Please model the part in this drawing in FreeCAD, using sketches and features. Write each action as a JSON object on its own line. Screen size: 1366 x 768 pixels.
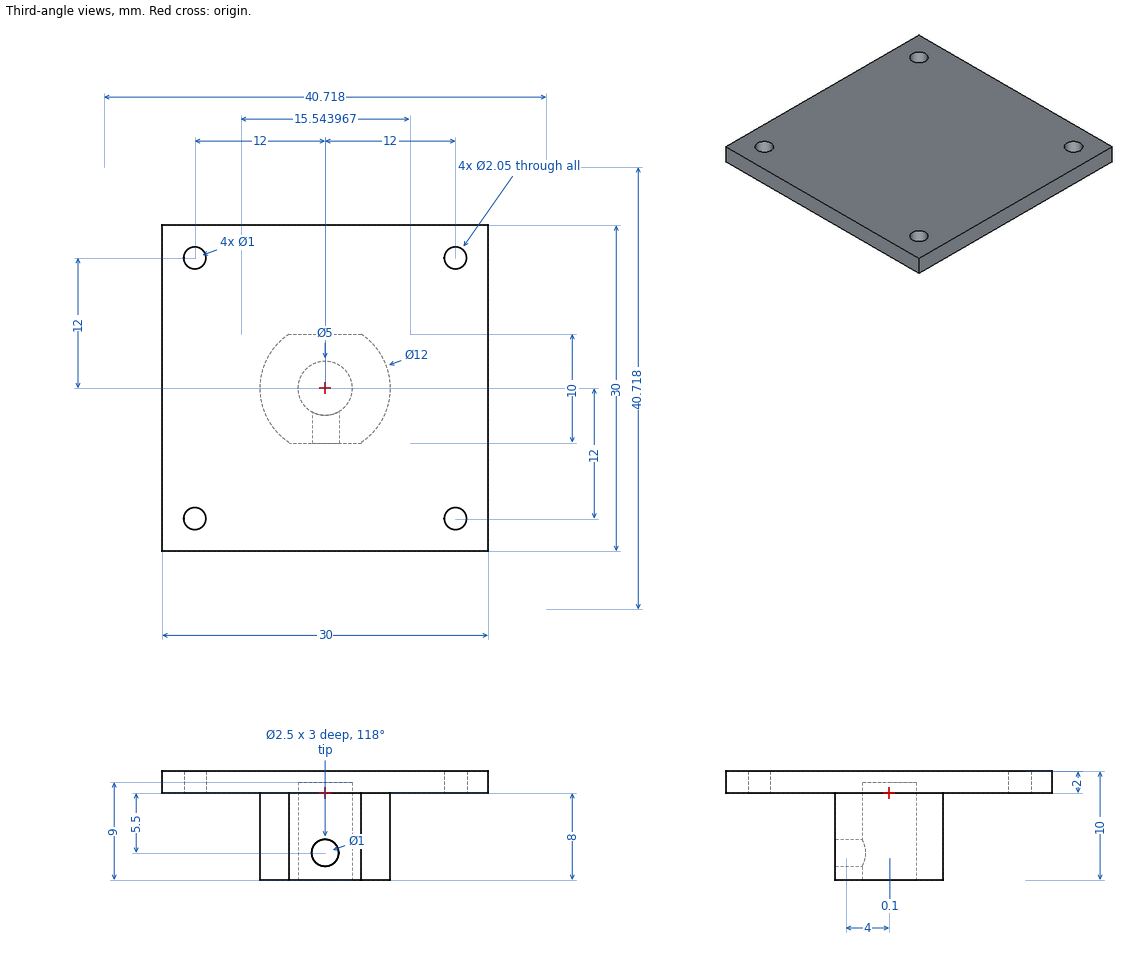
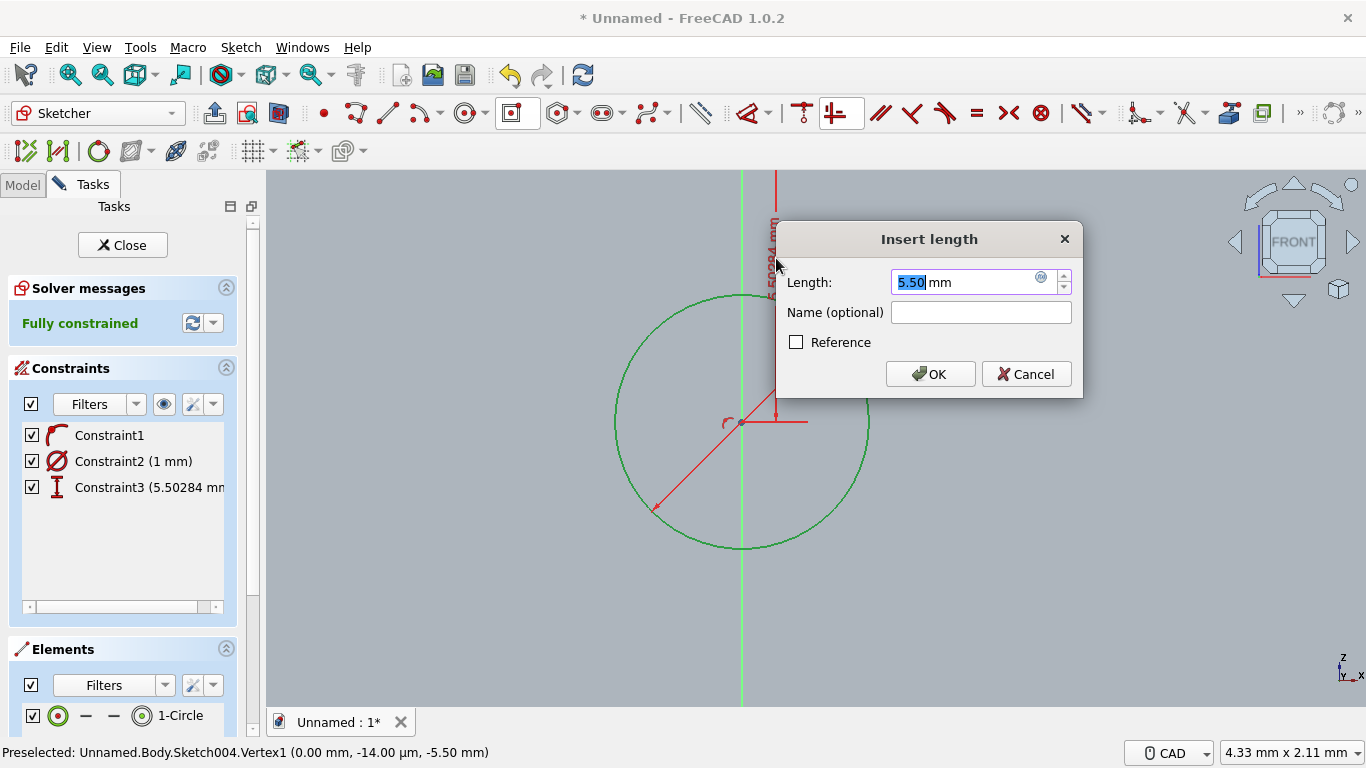
{"action": "type", "text": "5.5"}
{"action": "key", "text": "Return"}
{"action": "key", "text": "Escape"}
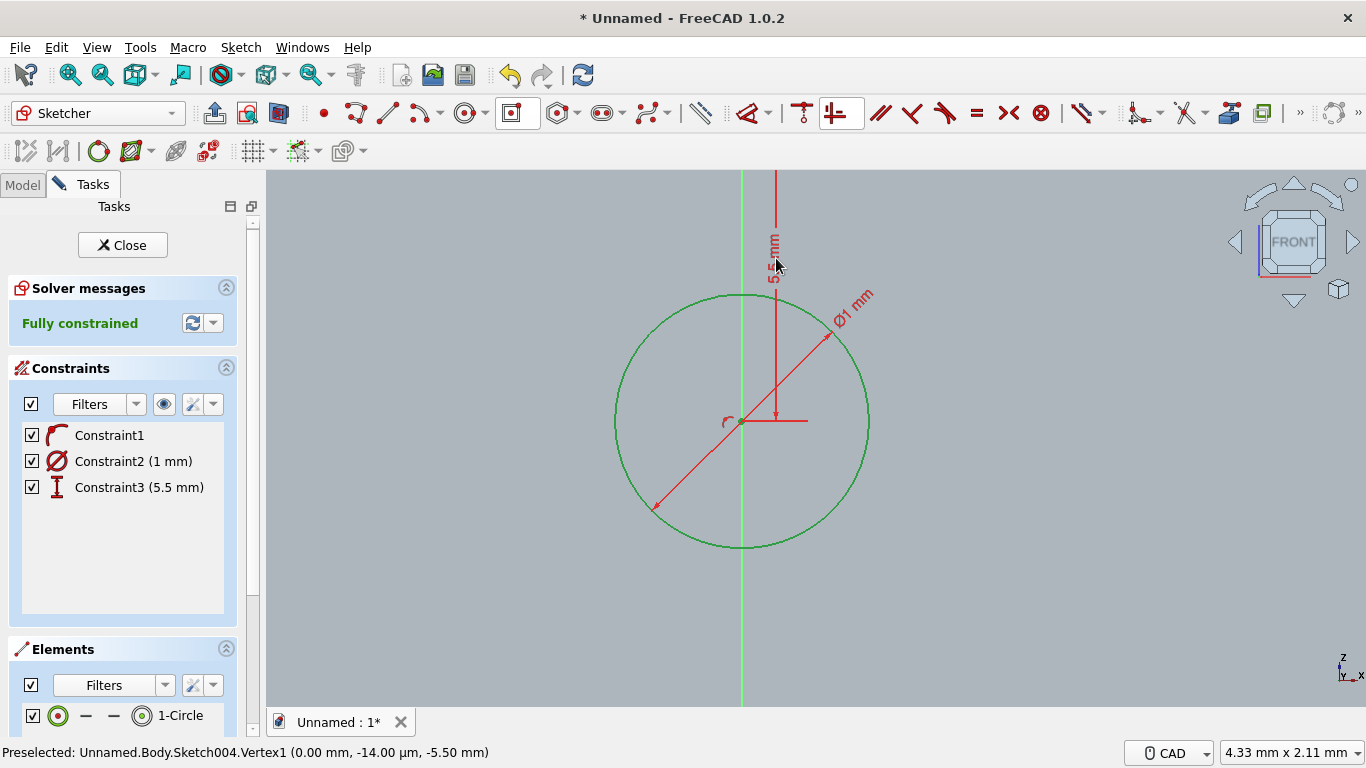
{"action": "left_click", "coordinate": [123, 245]}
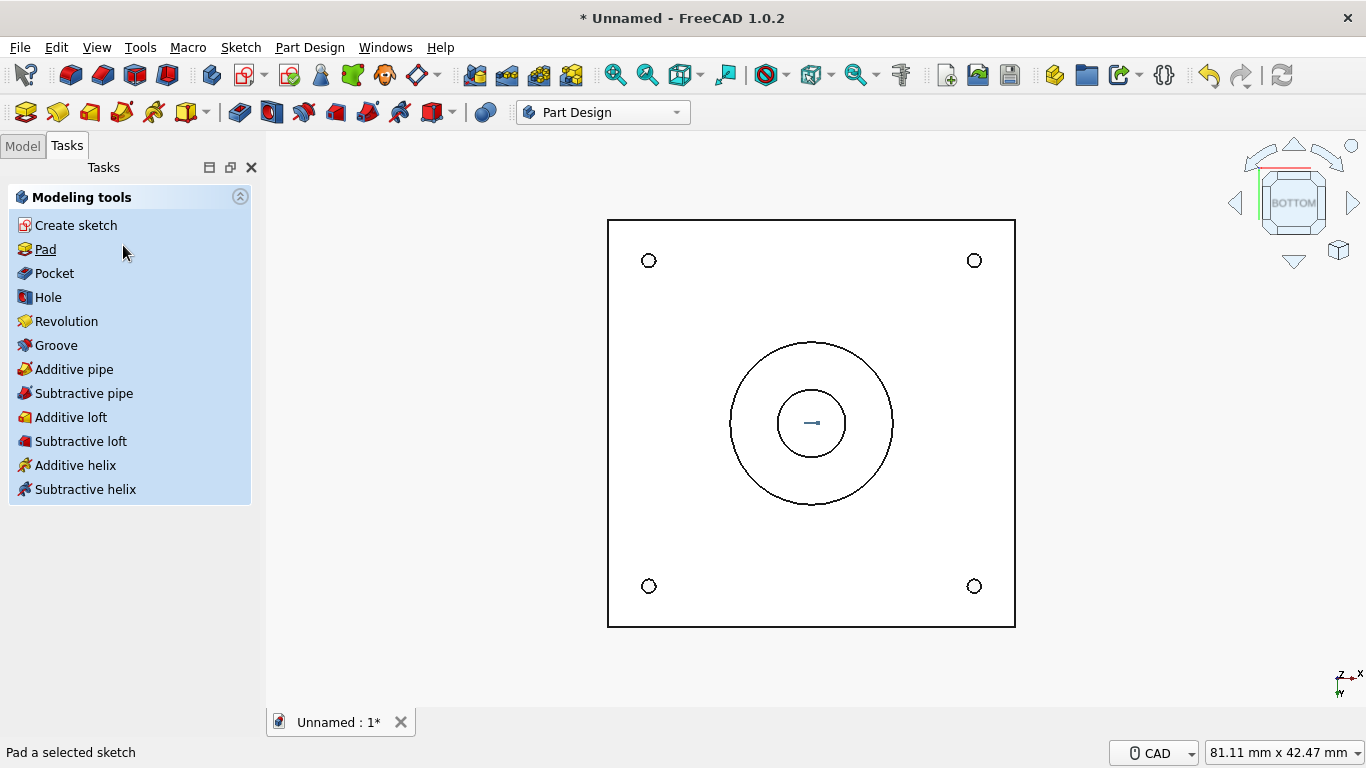
{"action": "left_click", "coordinate": [240, 112]}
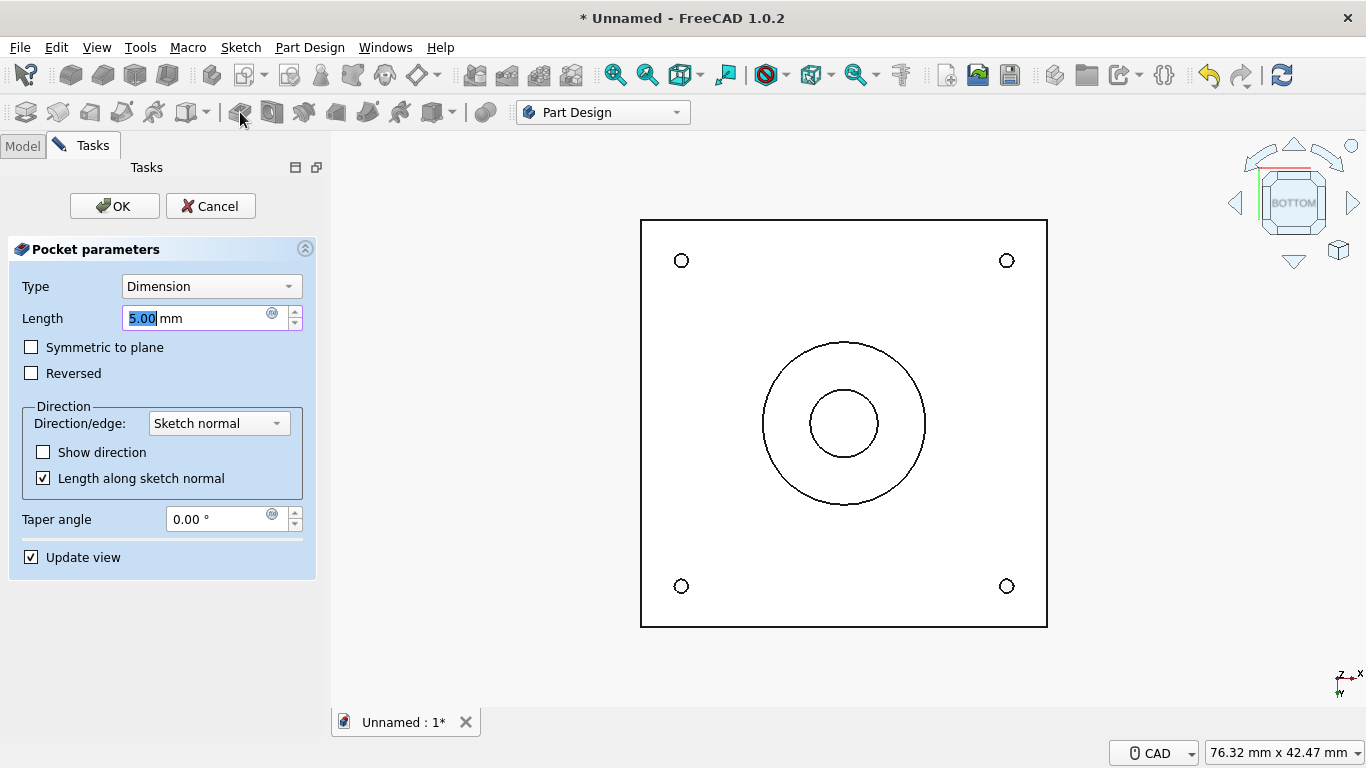
{"action": "left_click", "coordinate": [212, 286]}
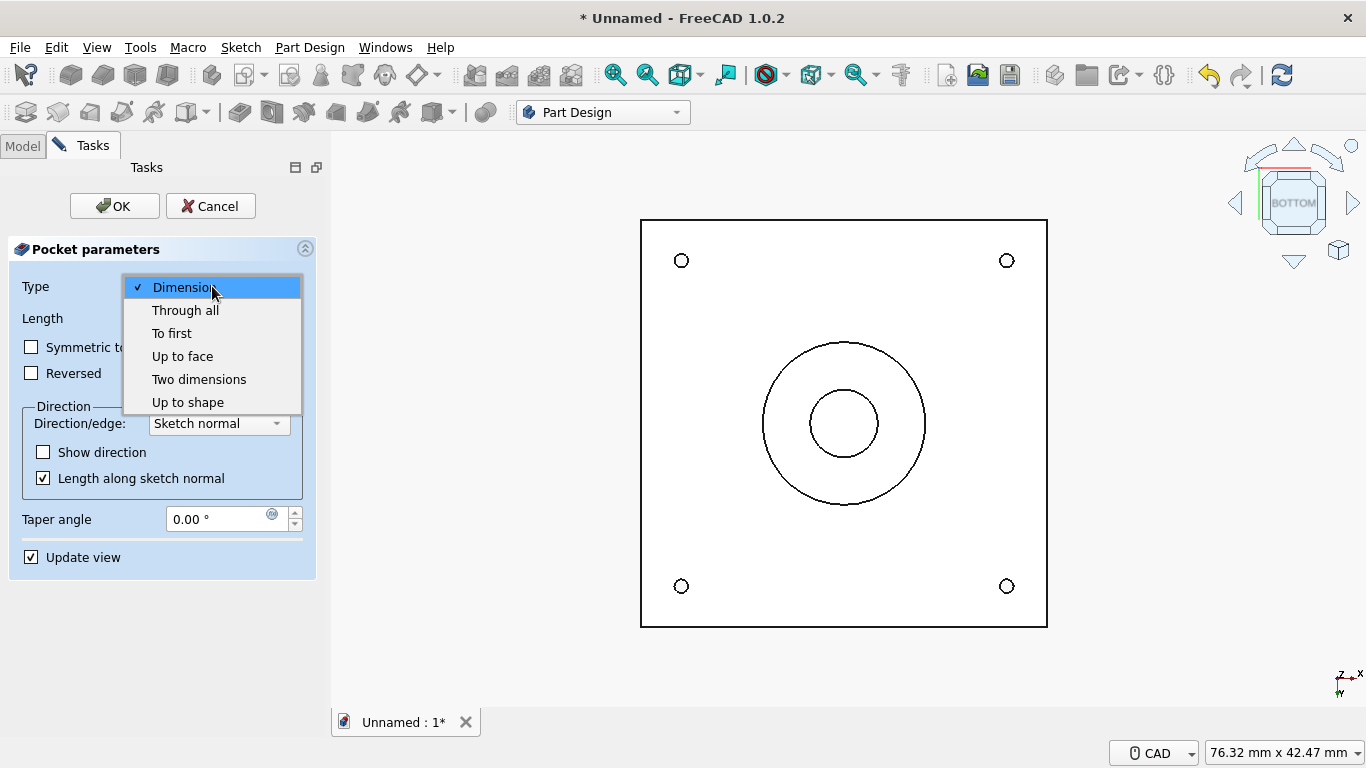
{"action": "left_click", "coordinate": [212, 380]}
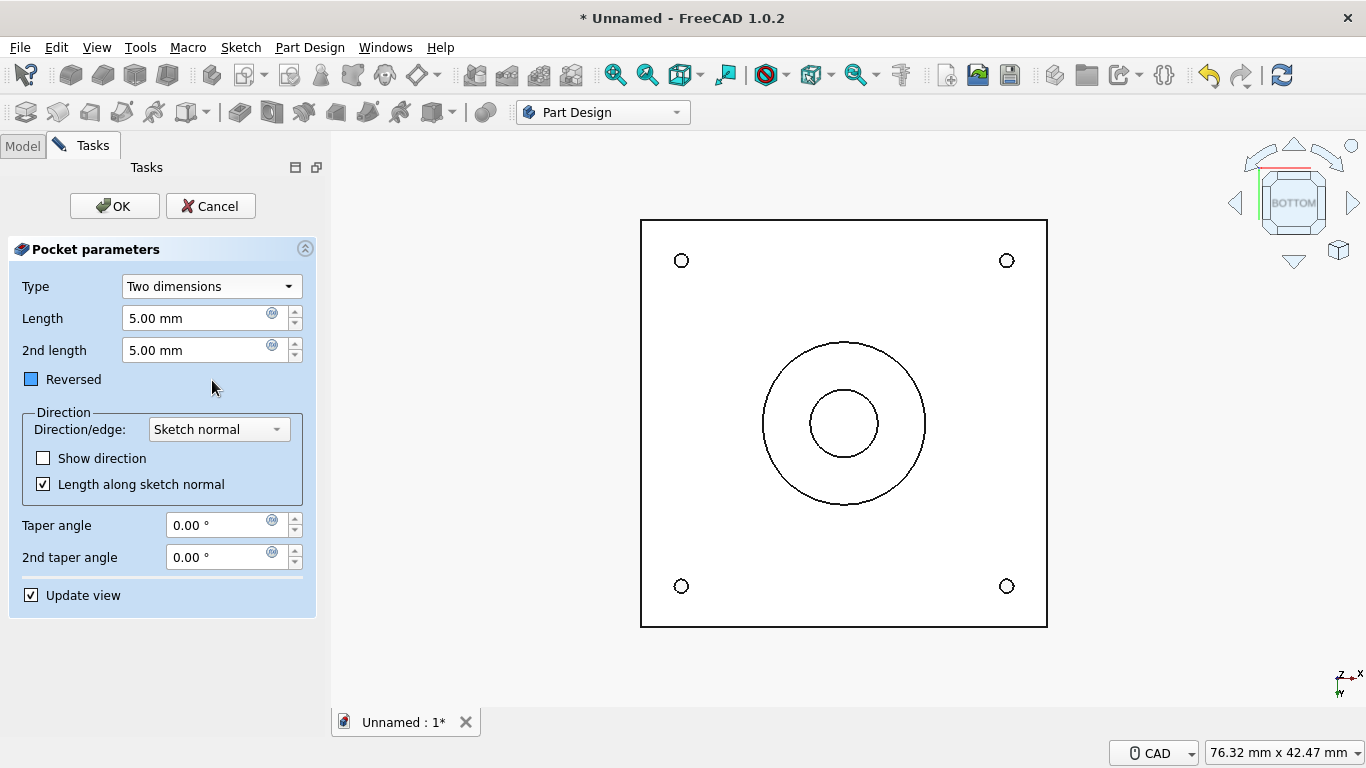
{"action": "triple_click", "coordinate": [204, 318]}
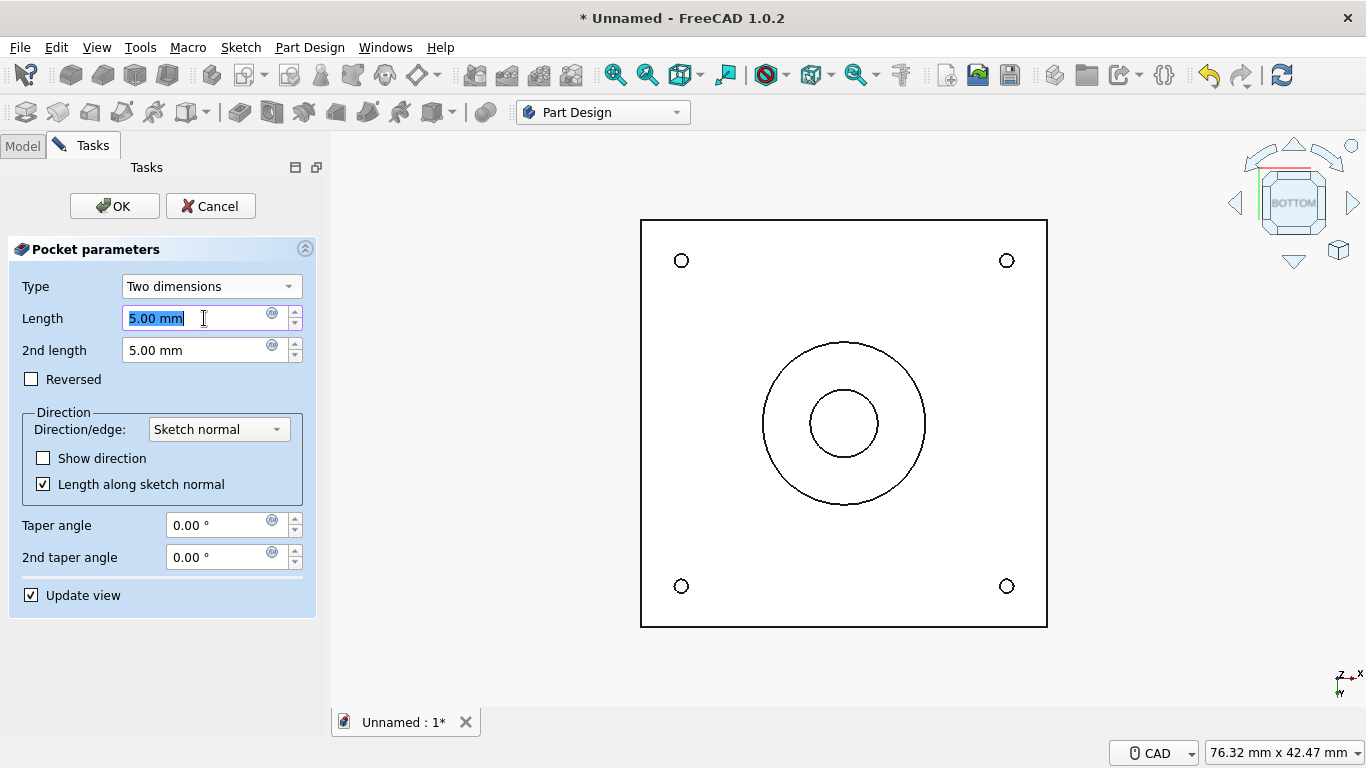
{"action": "type", "text": "0.1"}
{"action": "key", "text": "Tab"}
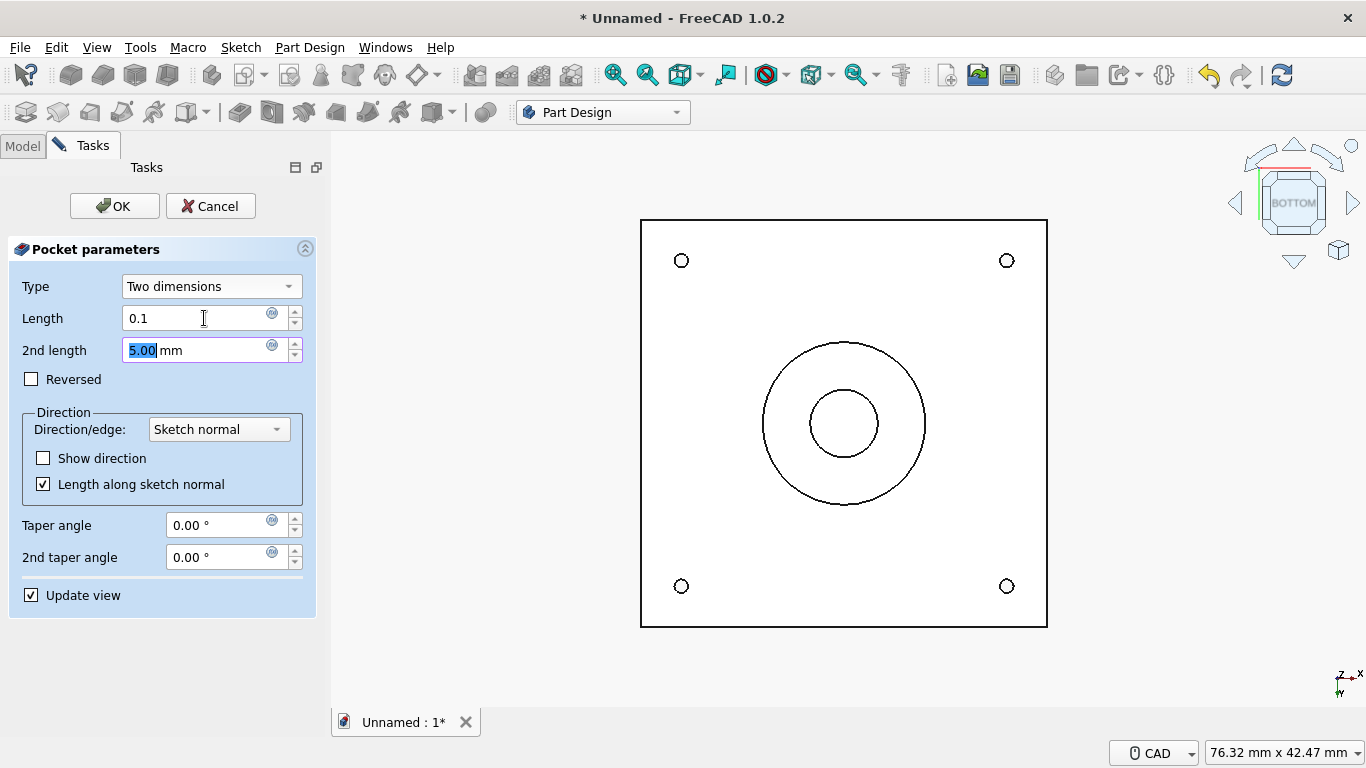
{"action": "type", "text": "4"}
{"action": "key", "text": "Tab"}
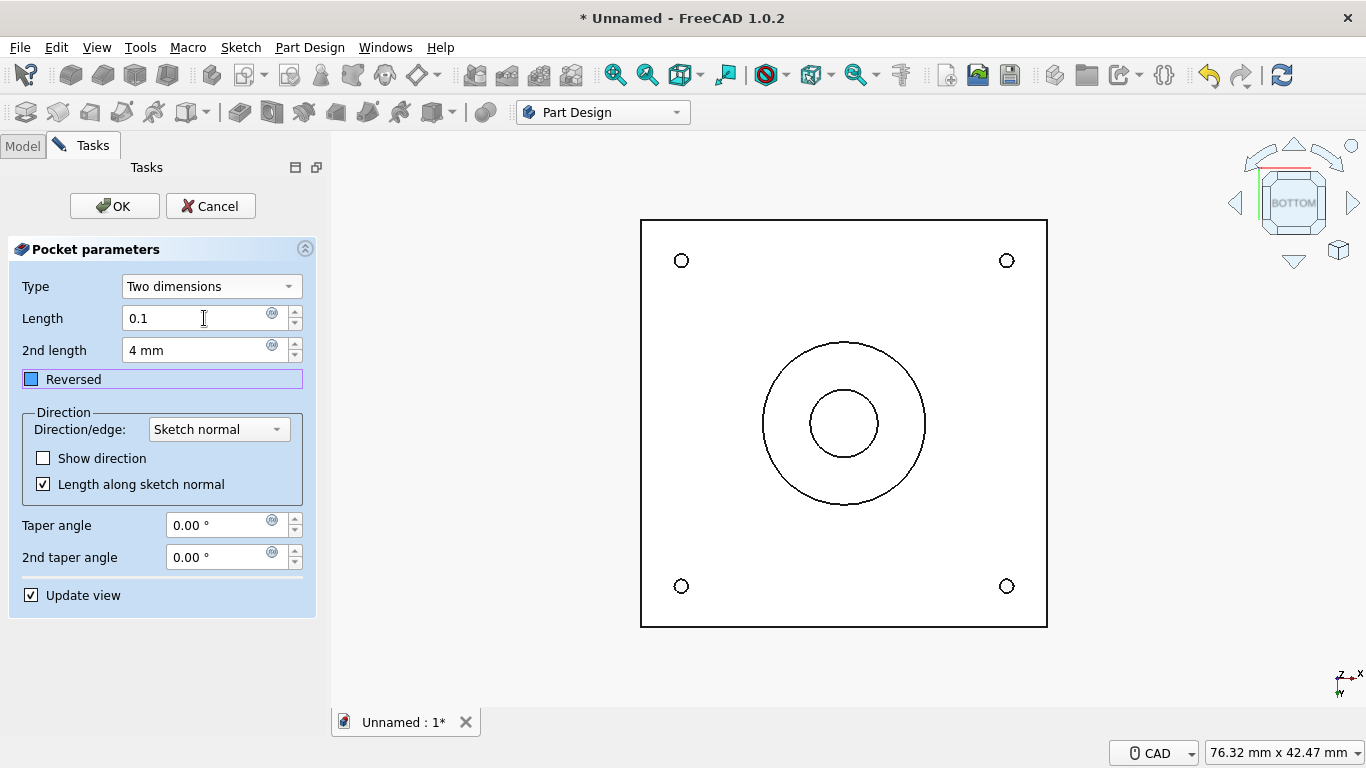
{"action": "left_click", "coordinate": [115, 206]}